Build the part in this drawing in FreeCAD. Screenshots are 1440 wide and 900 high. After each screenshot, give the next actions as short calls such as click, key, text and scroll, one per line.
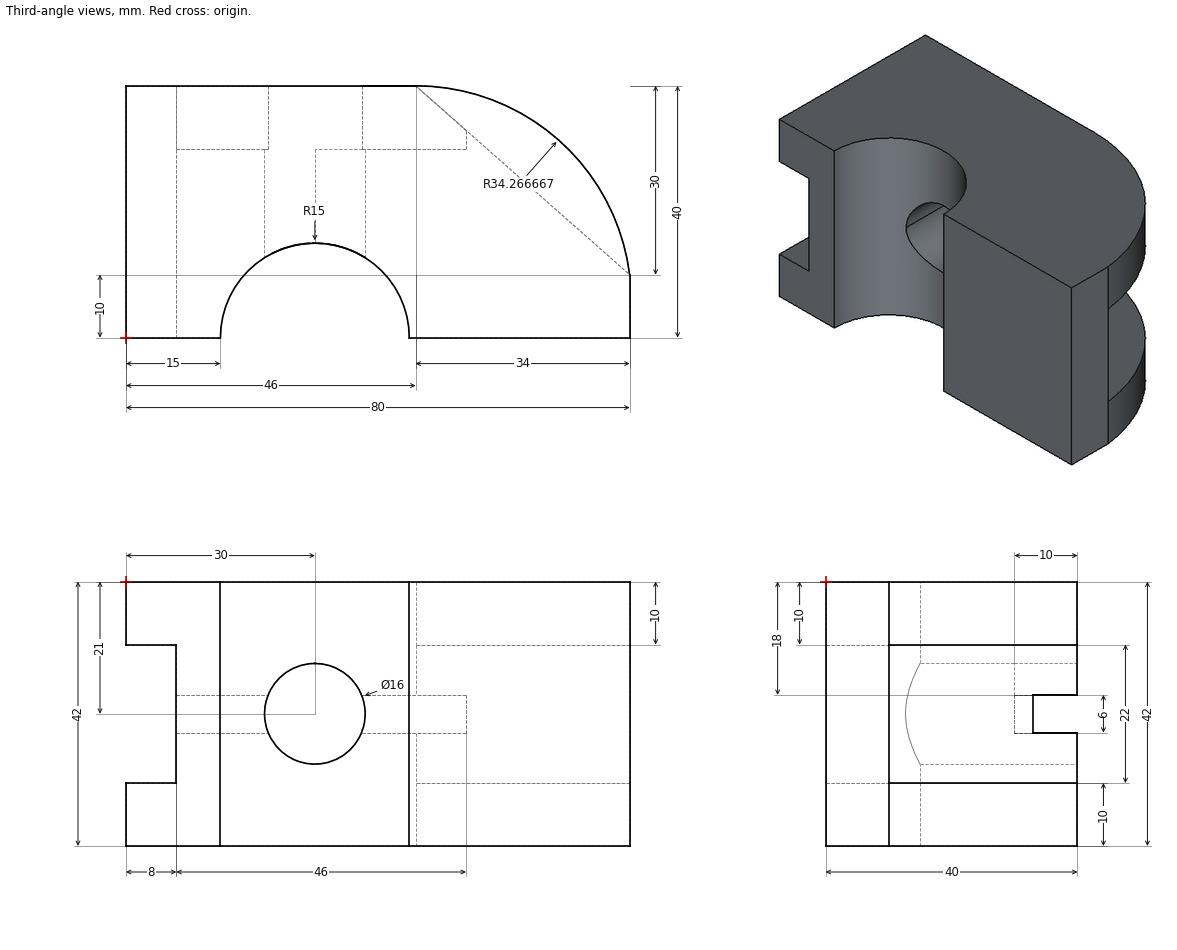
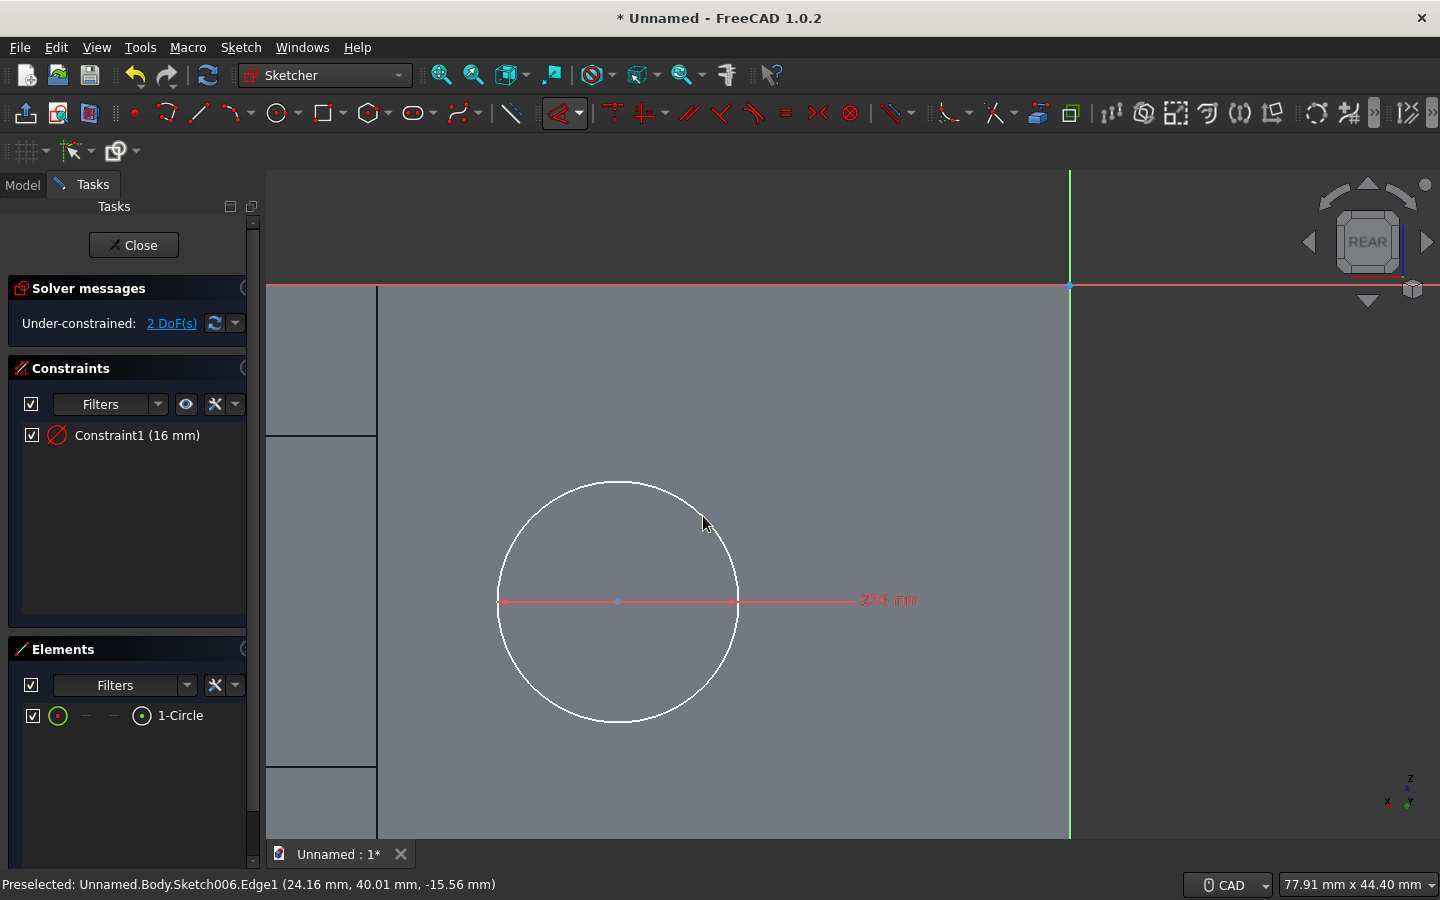
click(618, 602)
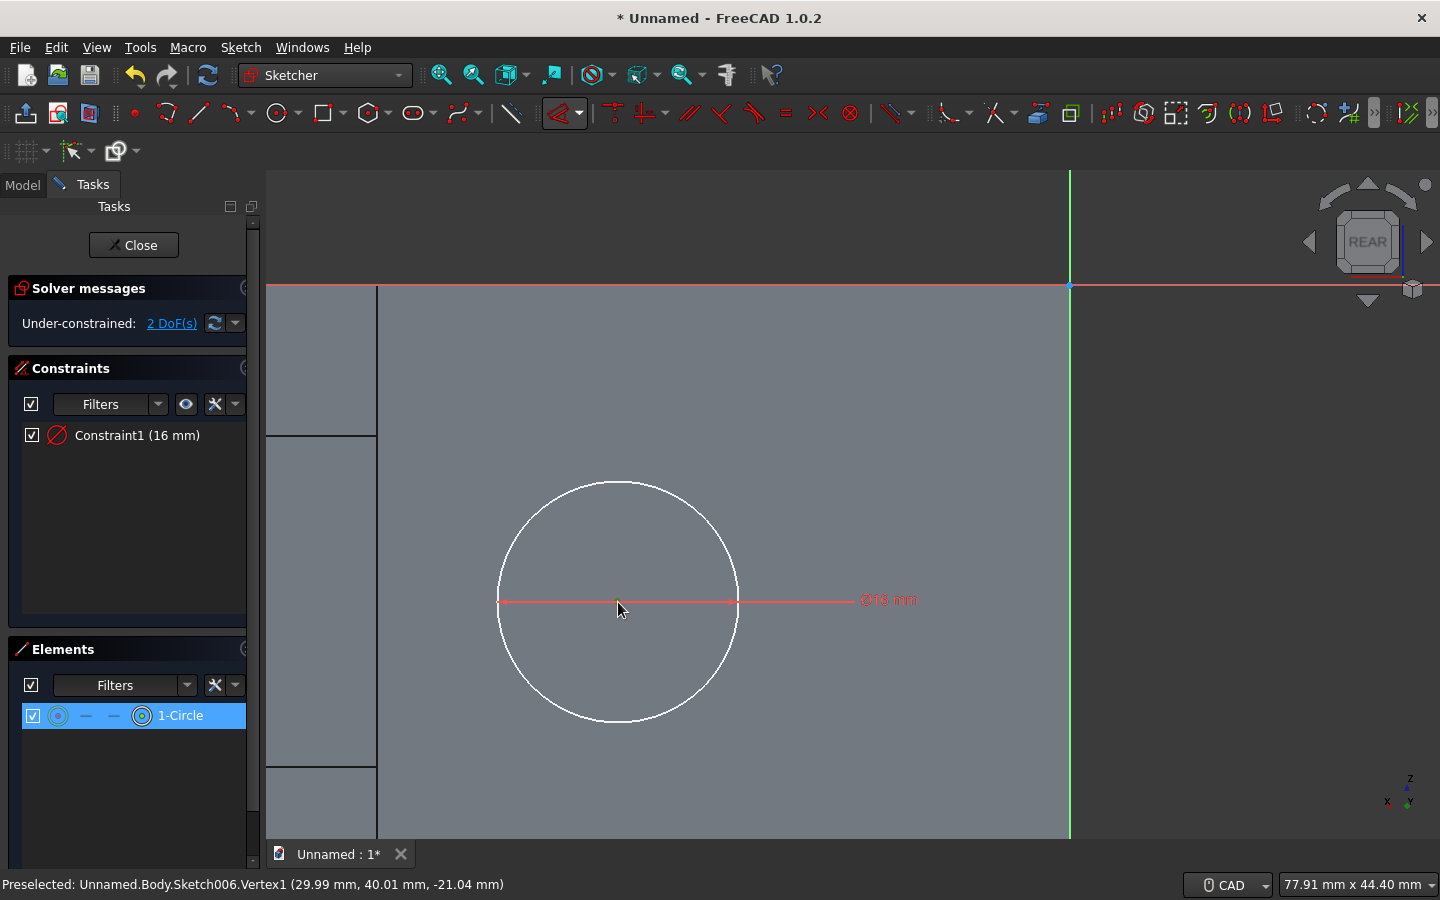
click(582, 114)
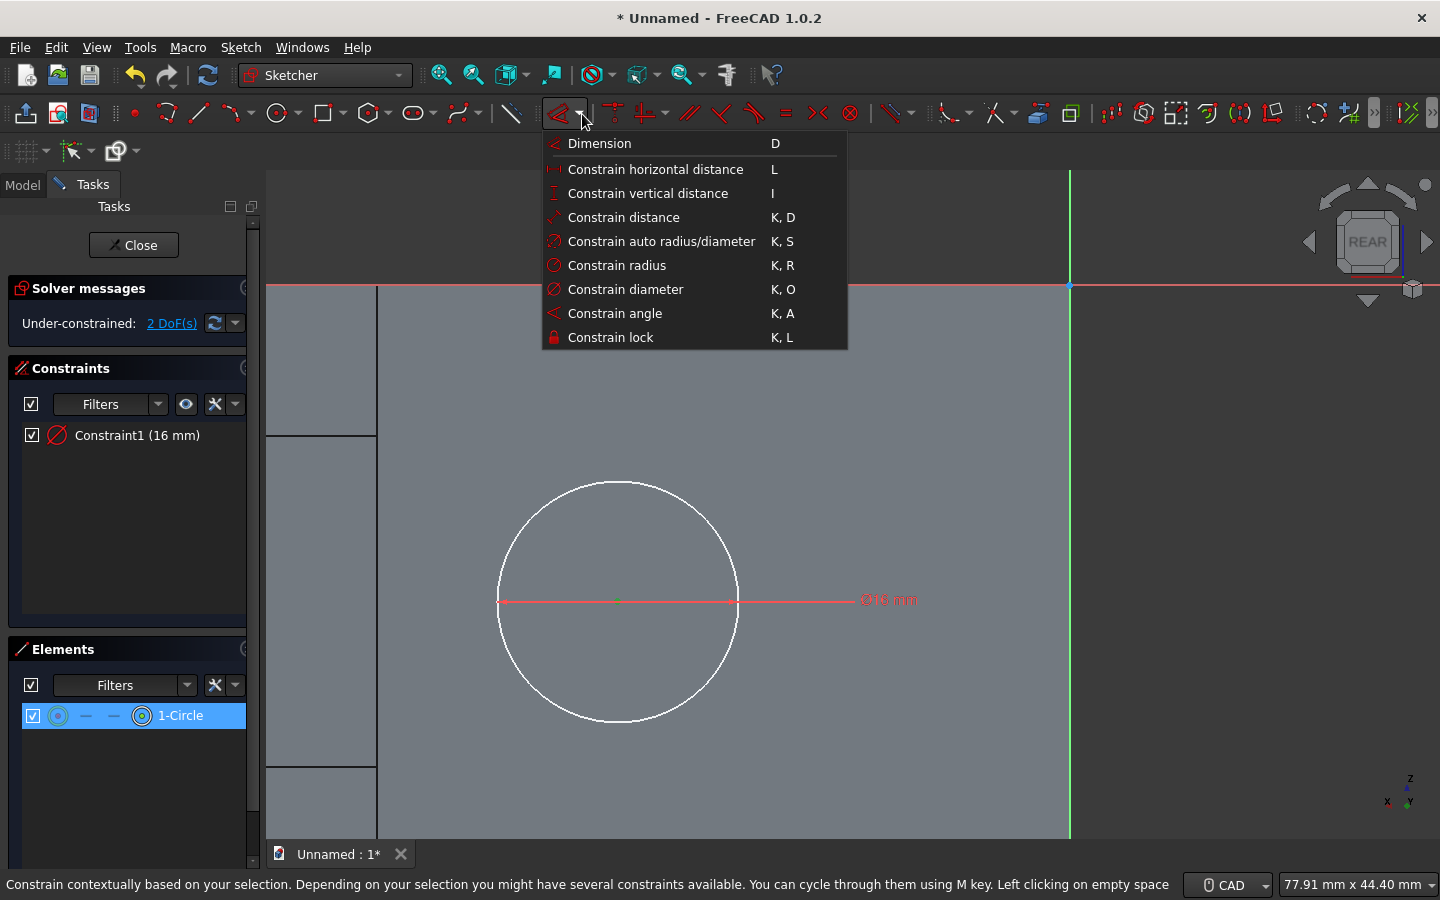
click(695, 169)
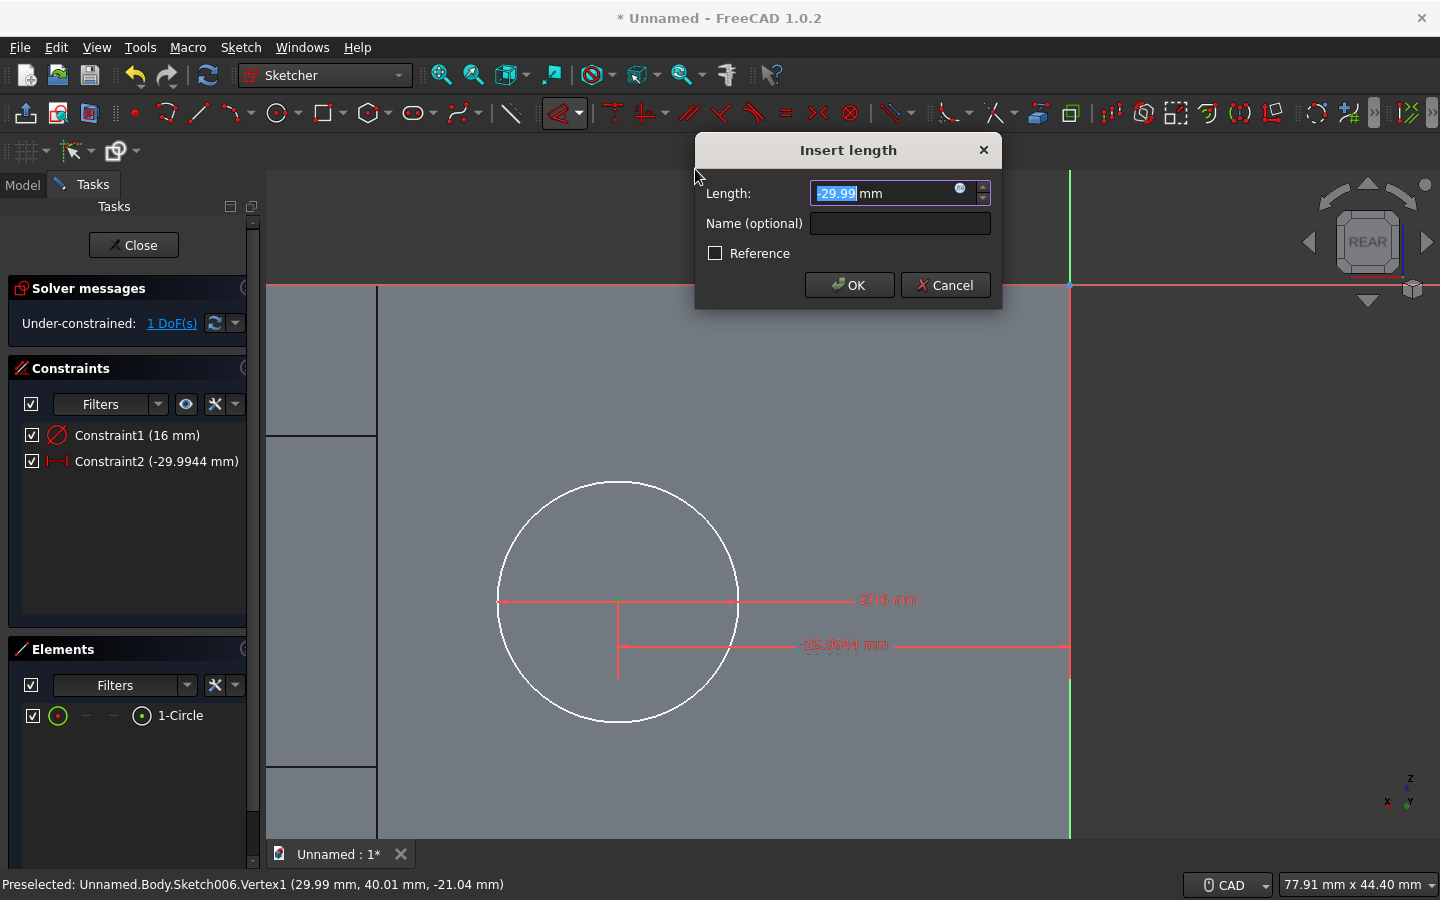
text(-30)
key(Return)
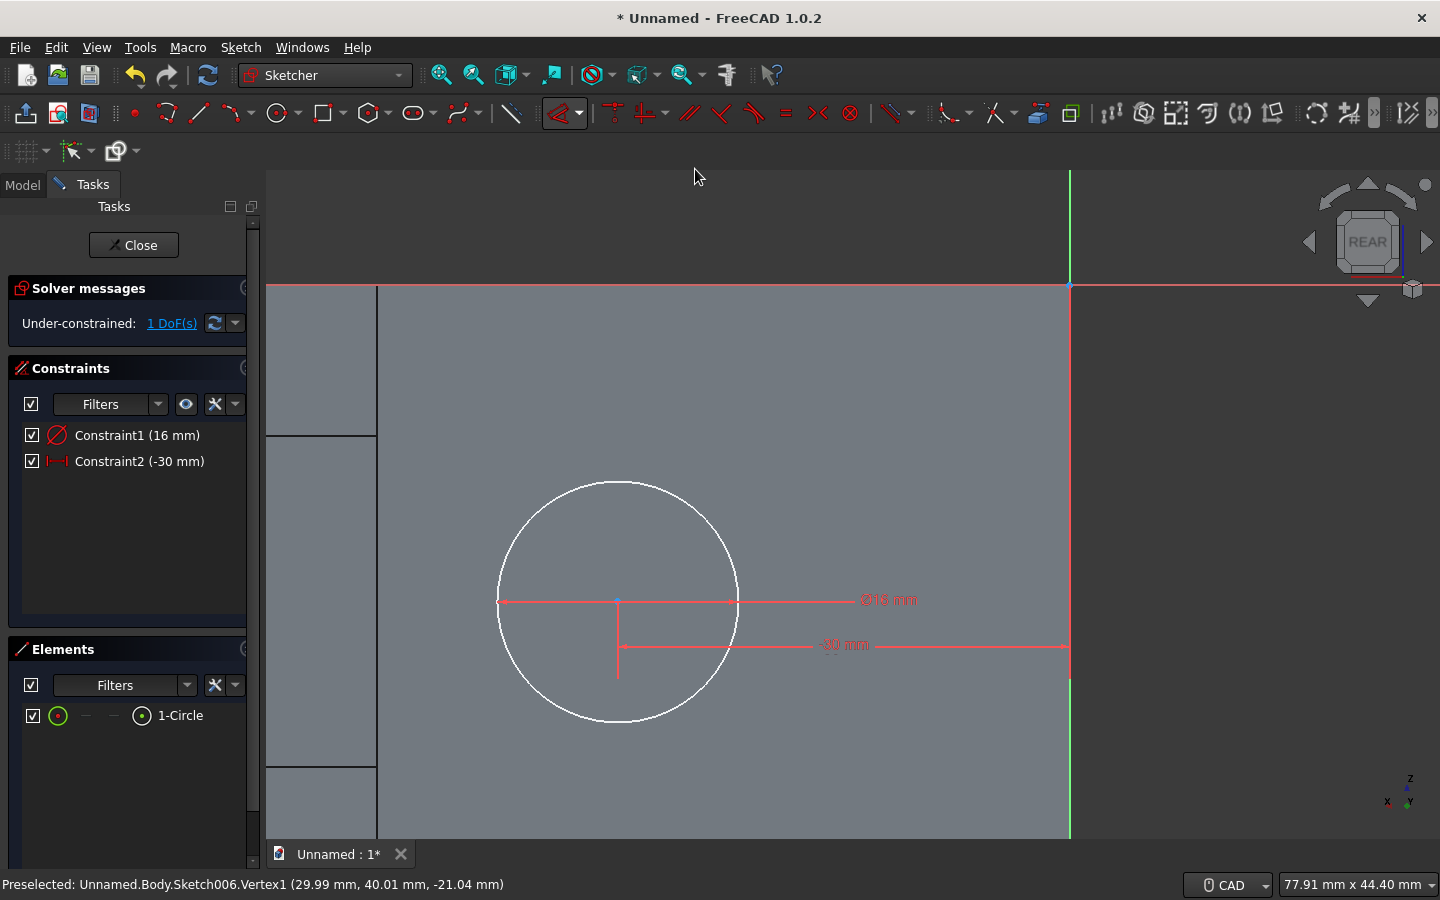
click(618, 602)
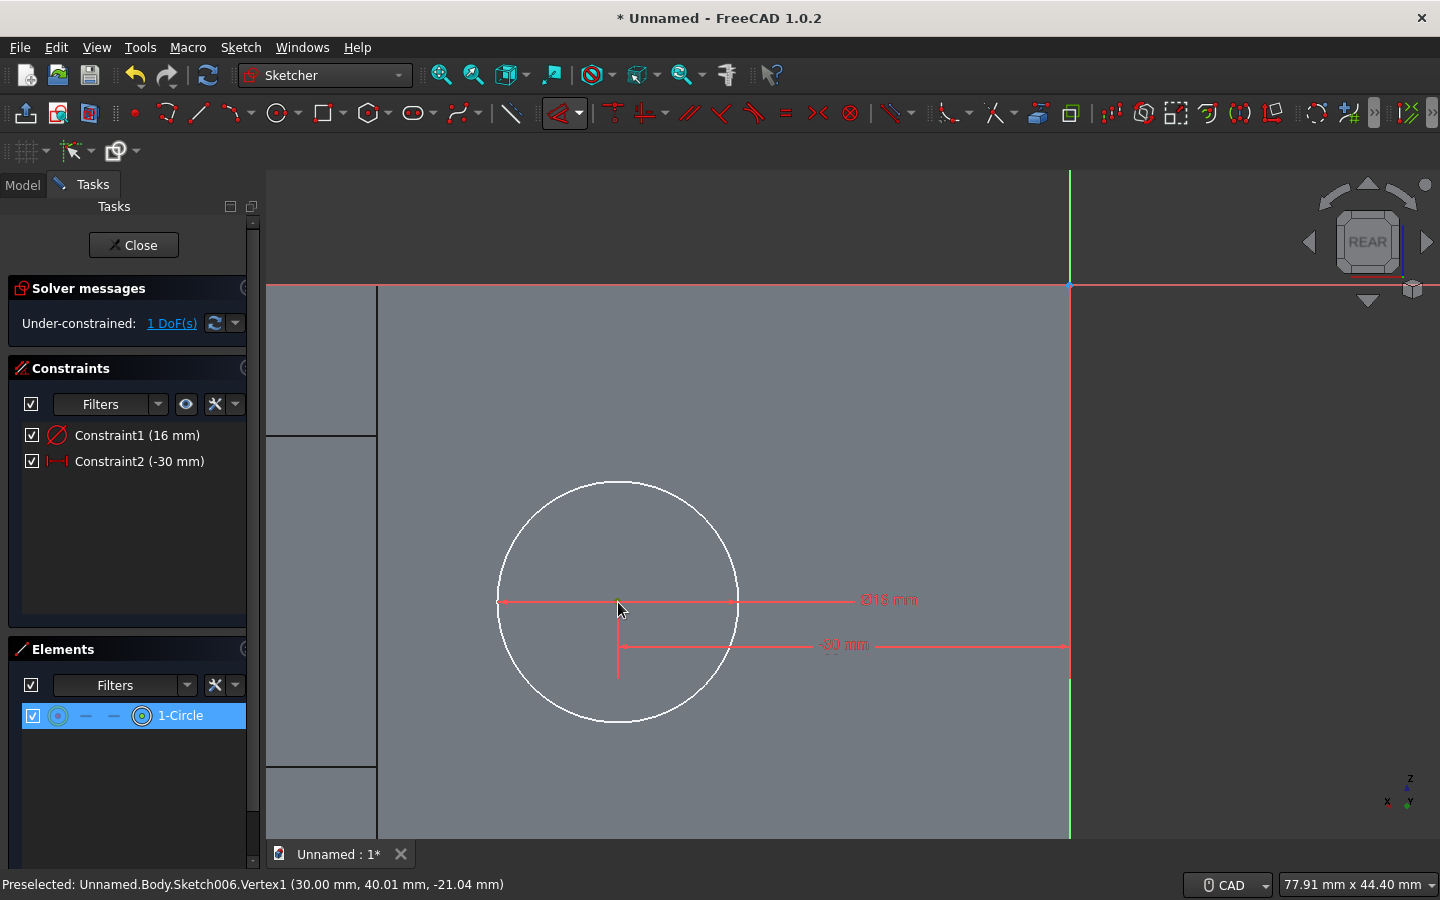
click(582, 114)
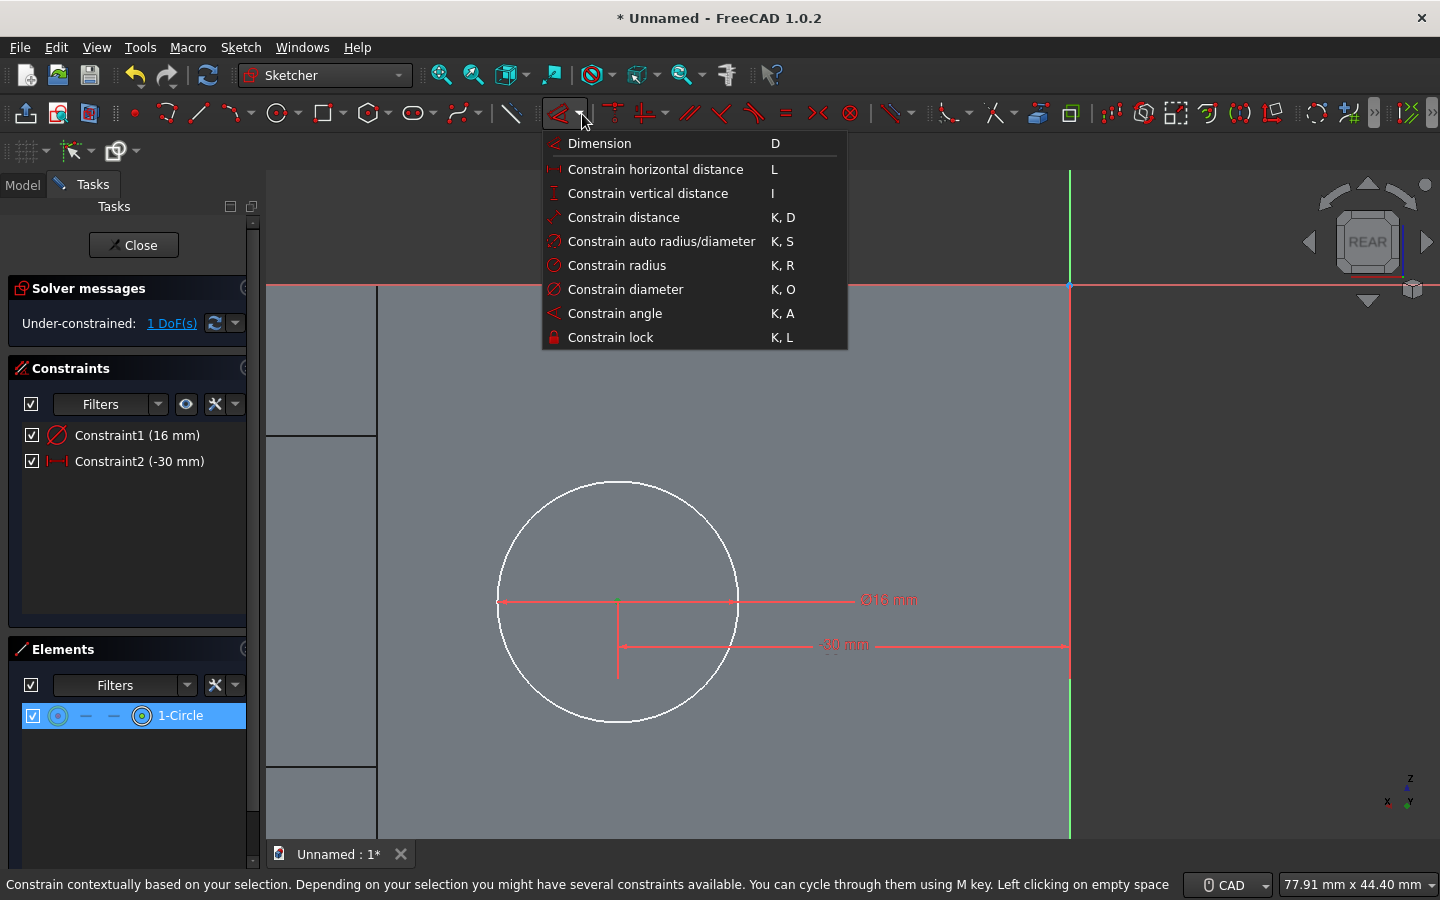
click(695, 193)